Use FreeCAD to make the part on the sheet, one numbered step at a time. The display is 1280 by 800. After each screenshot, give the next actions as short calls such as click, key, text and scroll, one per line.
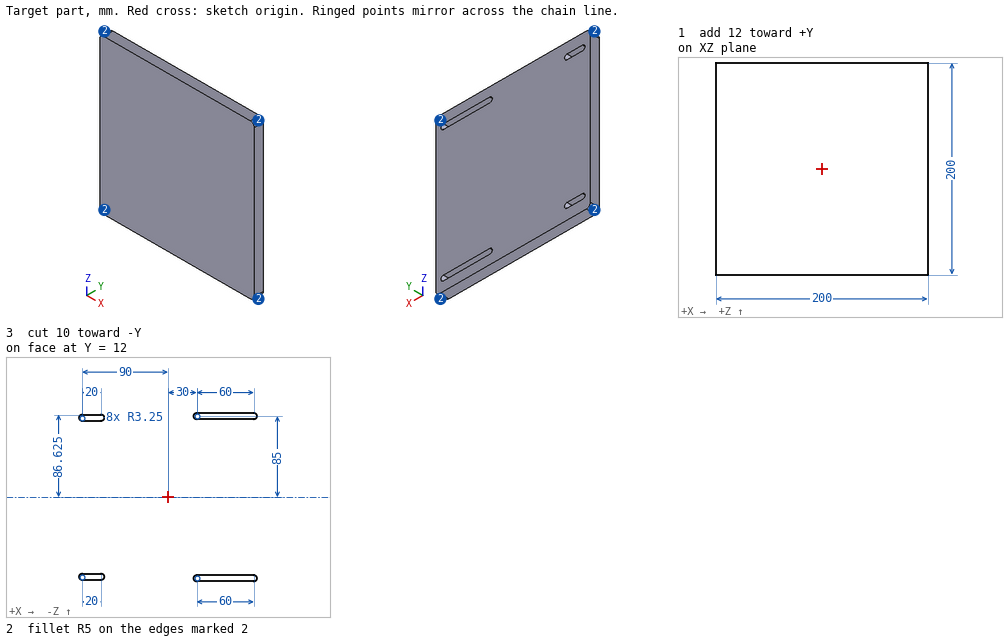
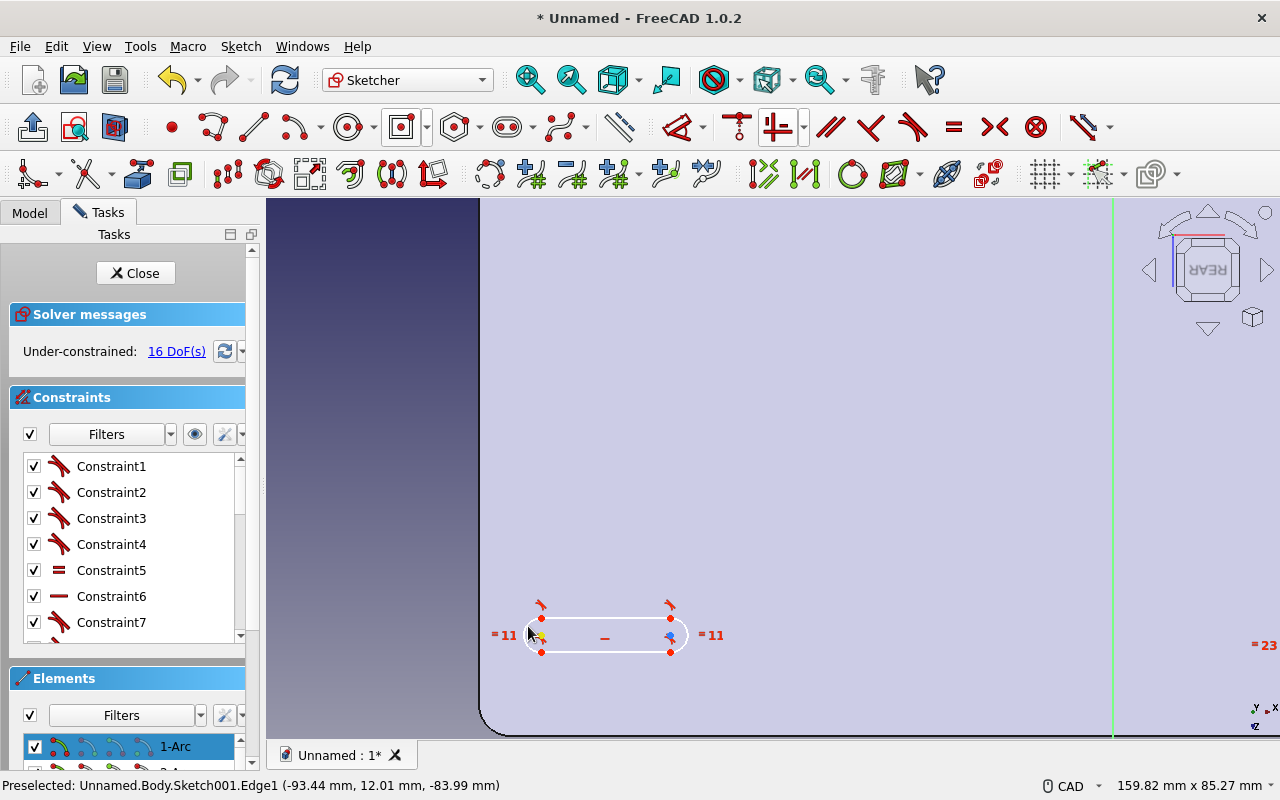
click(527, 625)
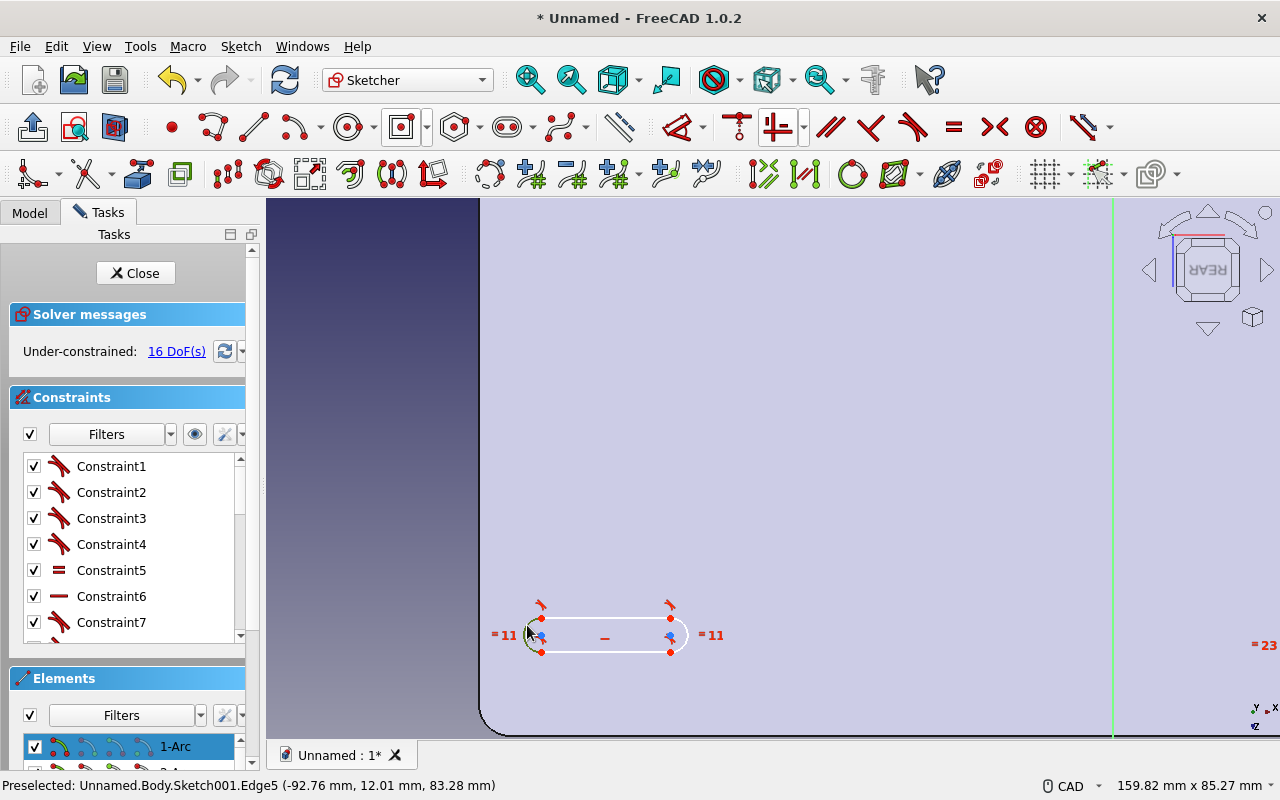
scroll(528, 627, down, 6)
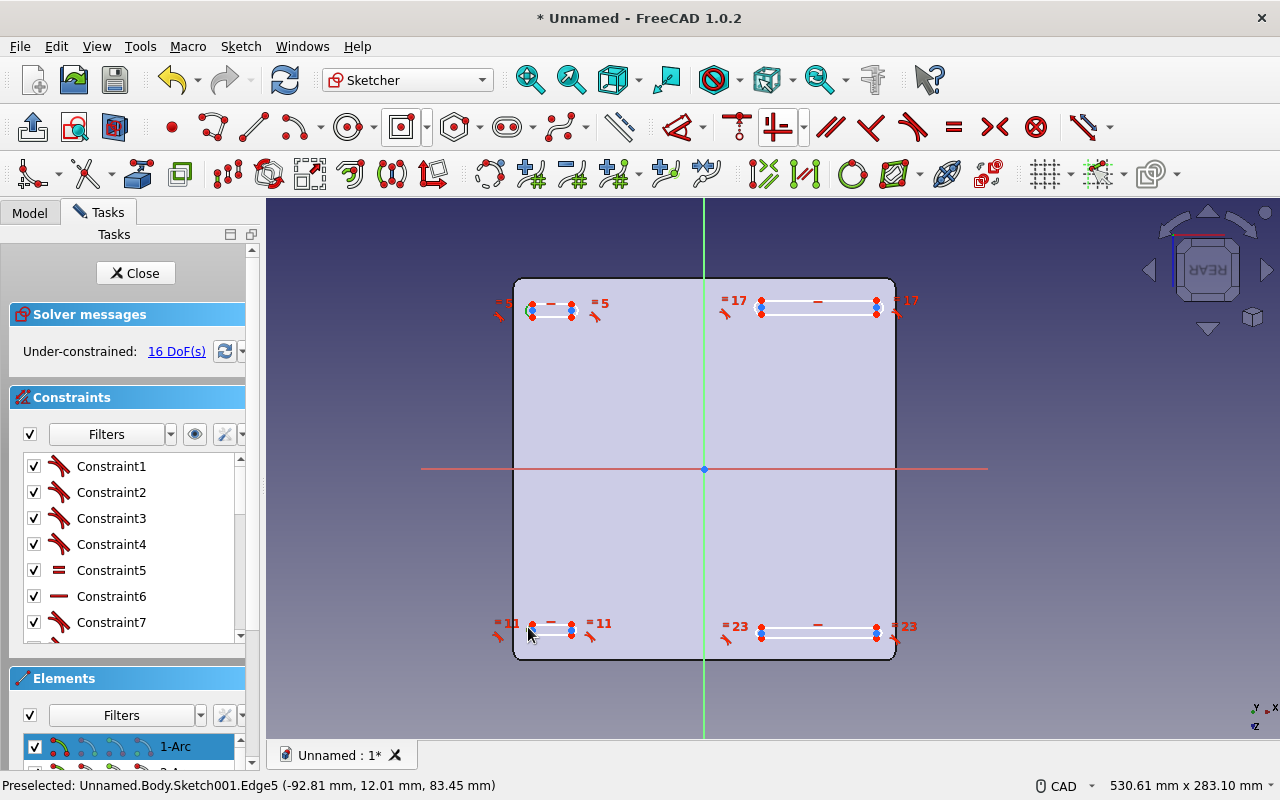
scroll(756, 304, up, 4)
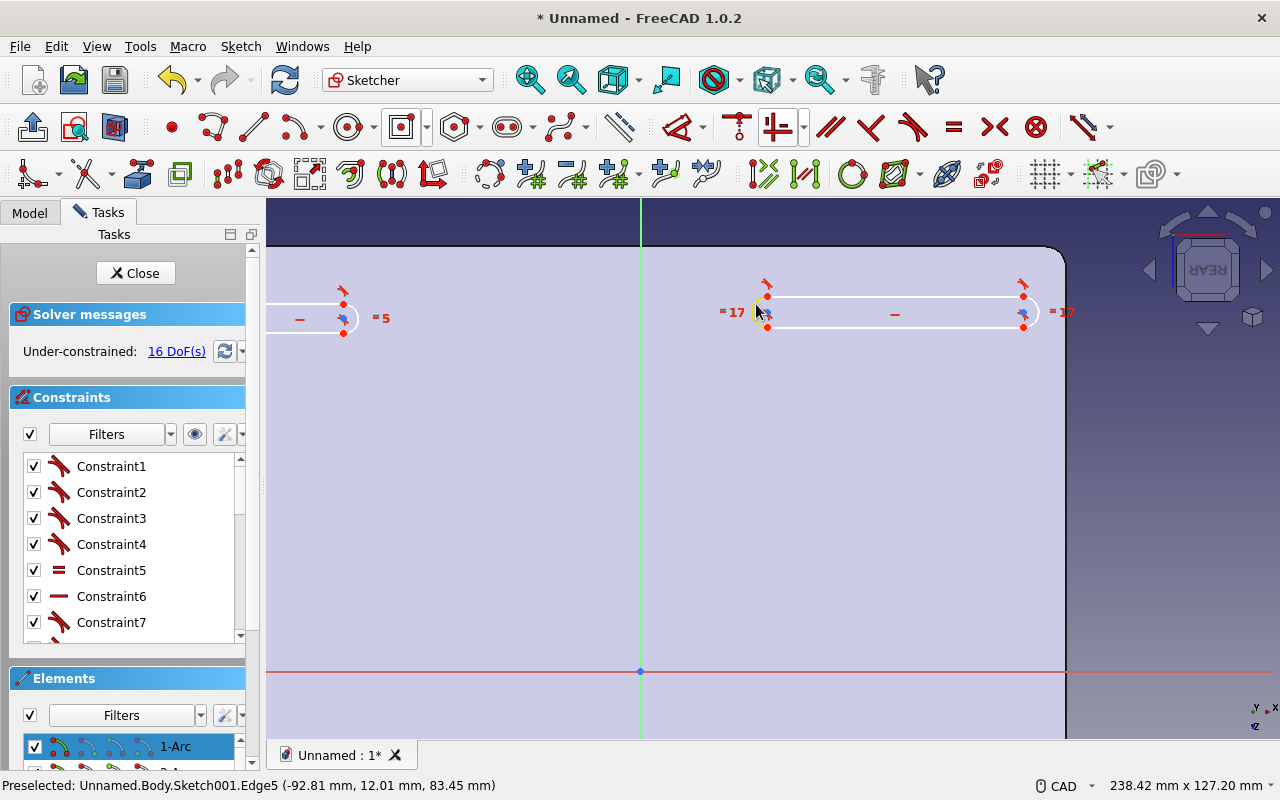
click(755, 303)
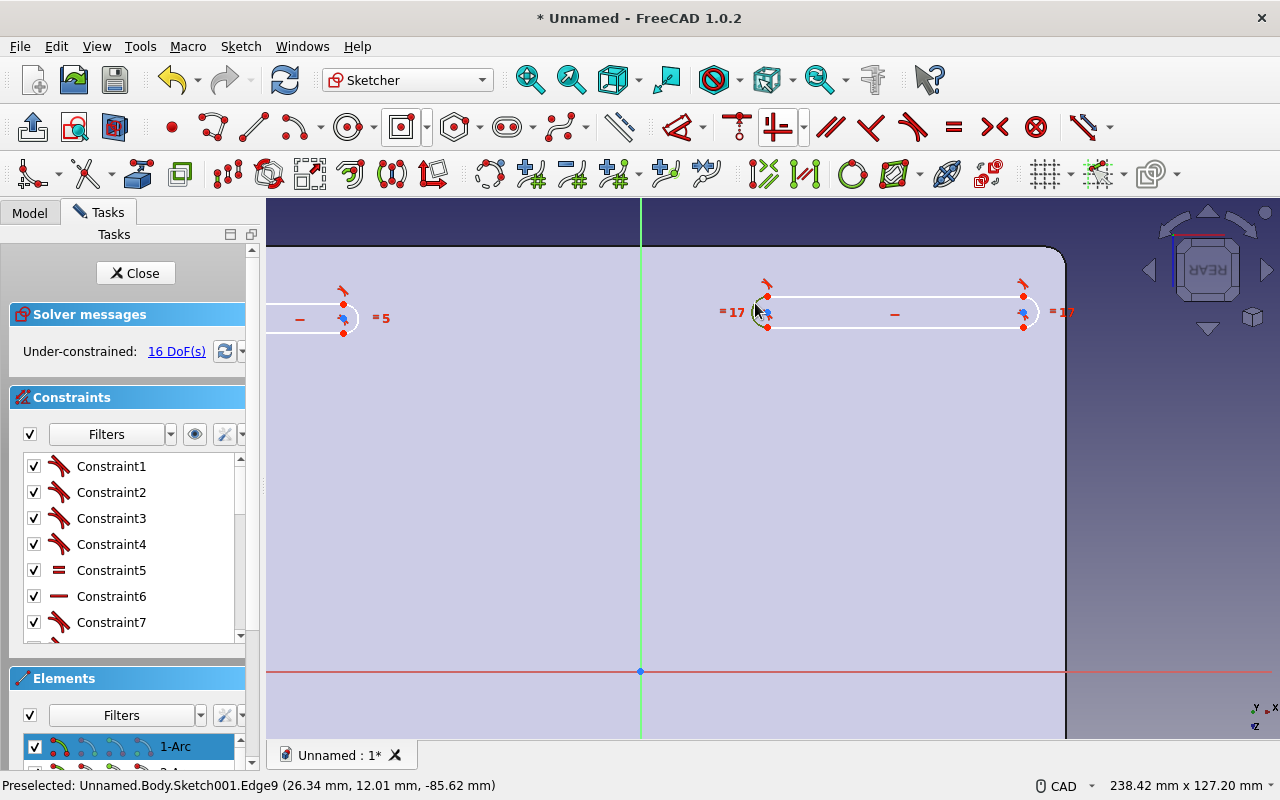
scroll(756, 303, down, 4)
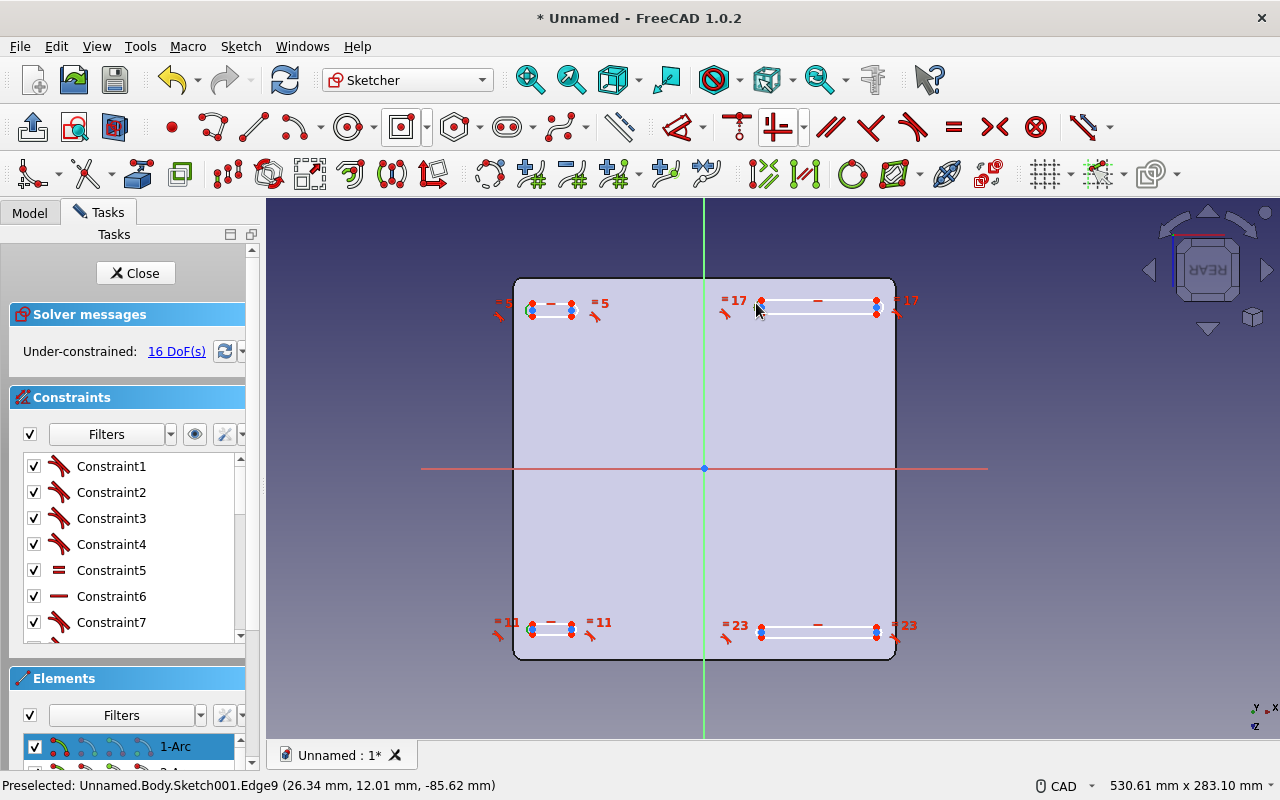
scroll(757, 629, up, 6)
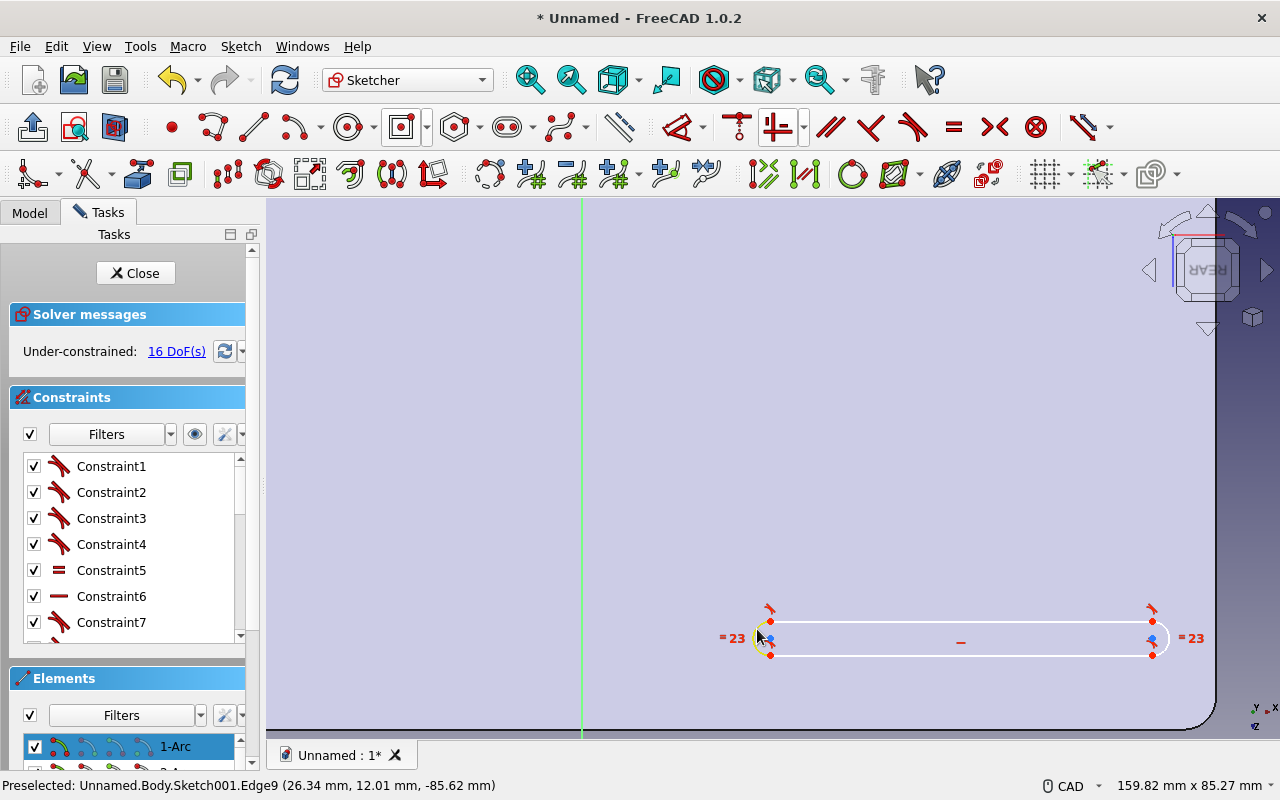
click(757, 629)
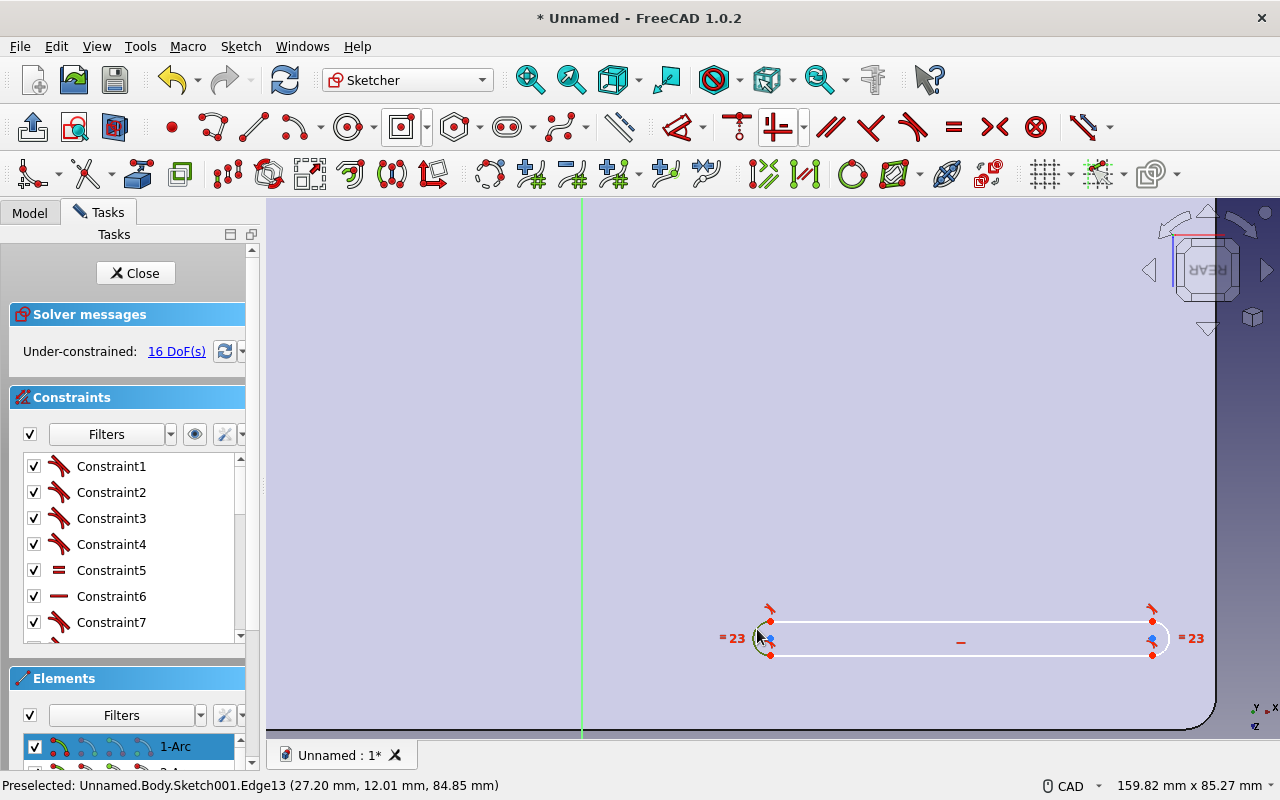
click(954, 128)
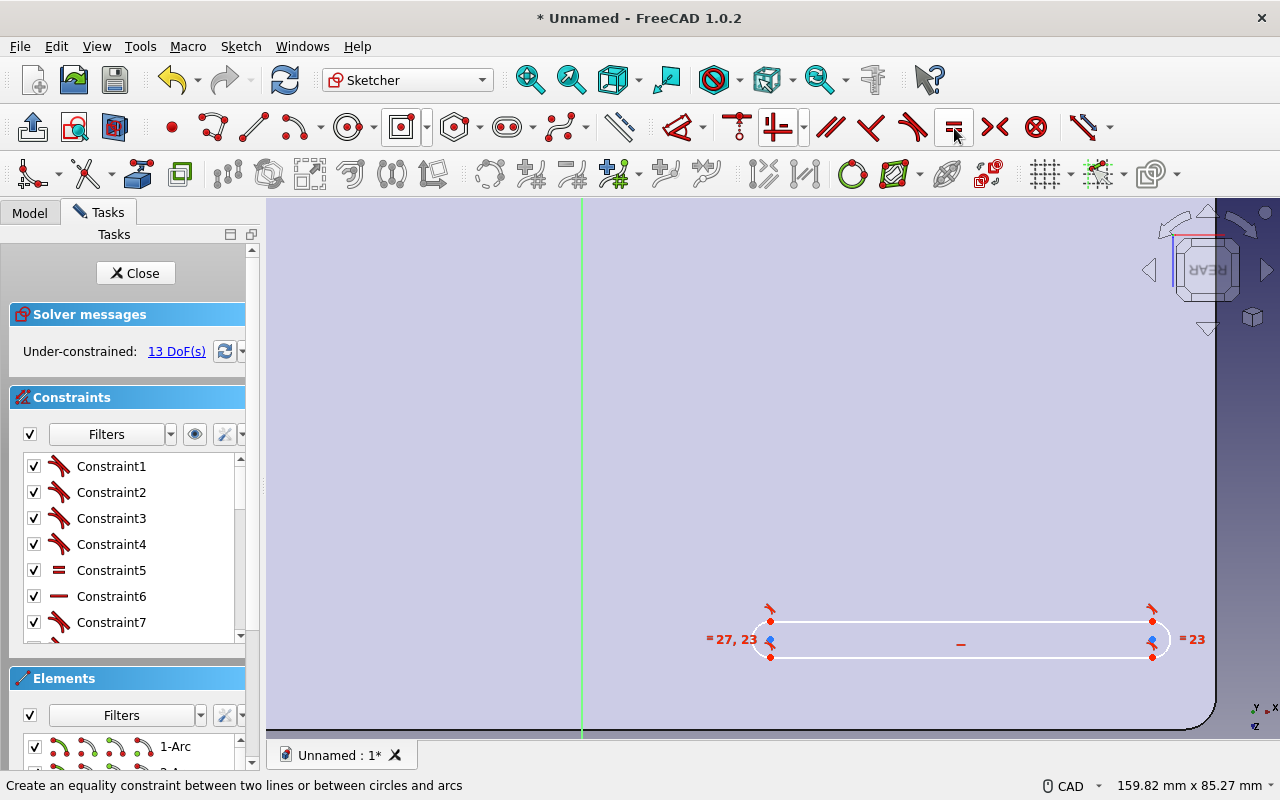
scroll(757, 629, down, 6)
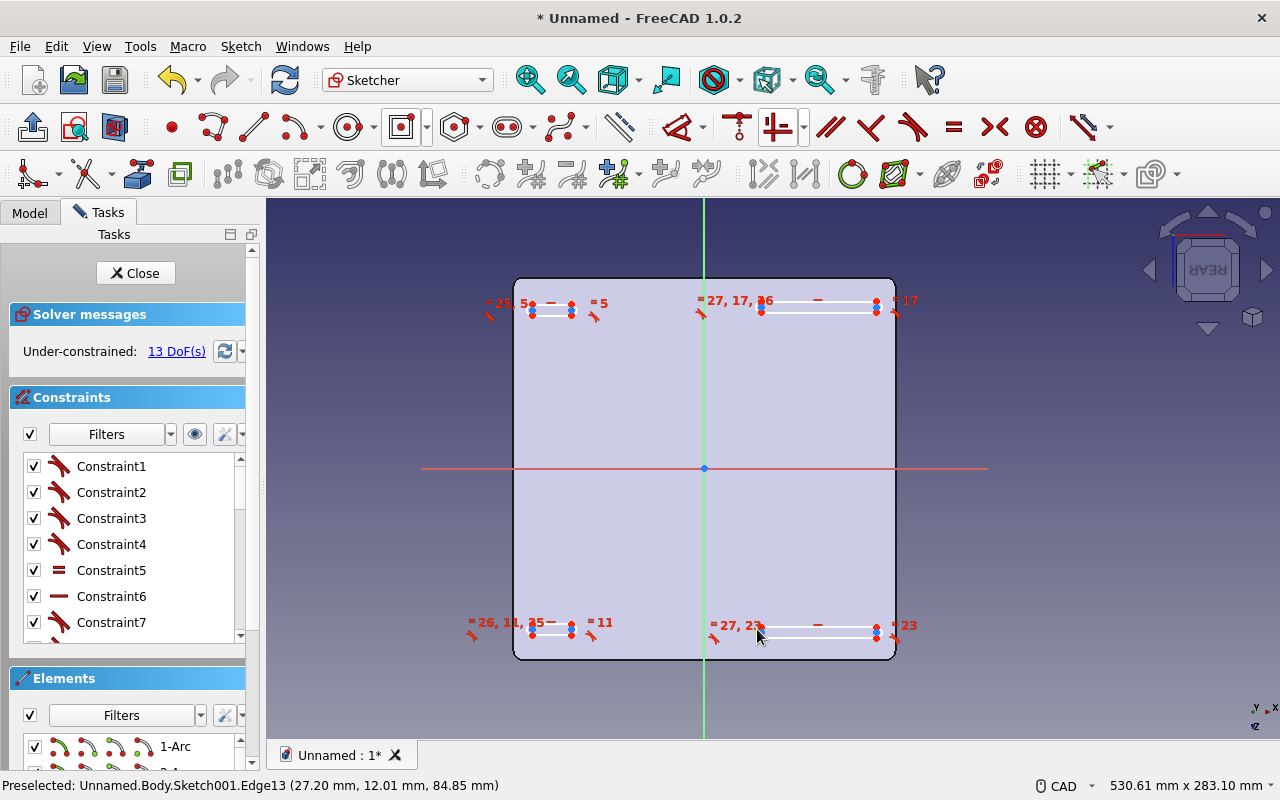
scroll(532, 310, up, 5)